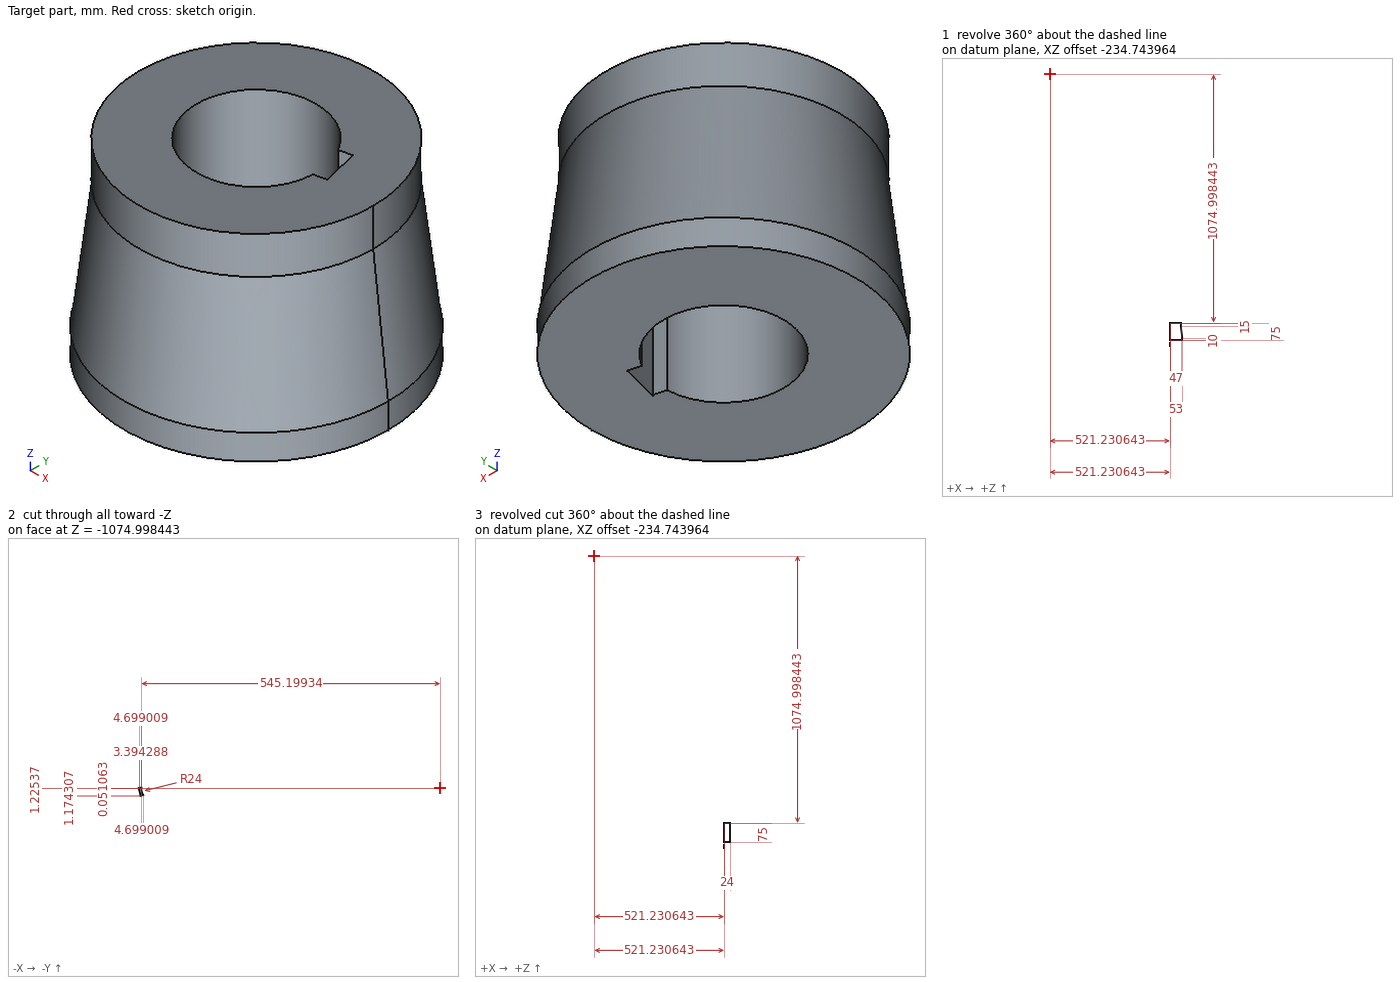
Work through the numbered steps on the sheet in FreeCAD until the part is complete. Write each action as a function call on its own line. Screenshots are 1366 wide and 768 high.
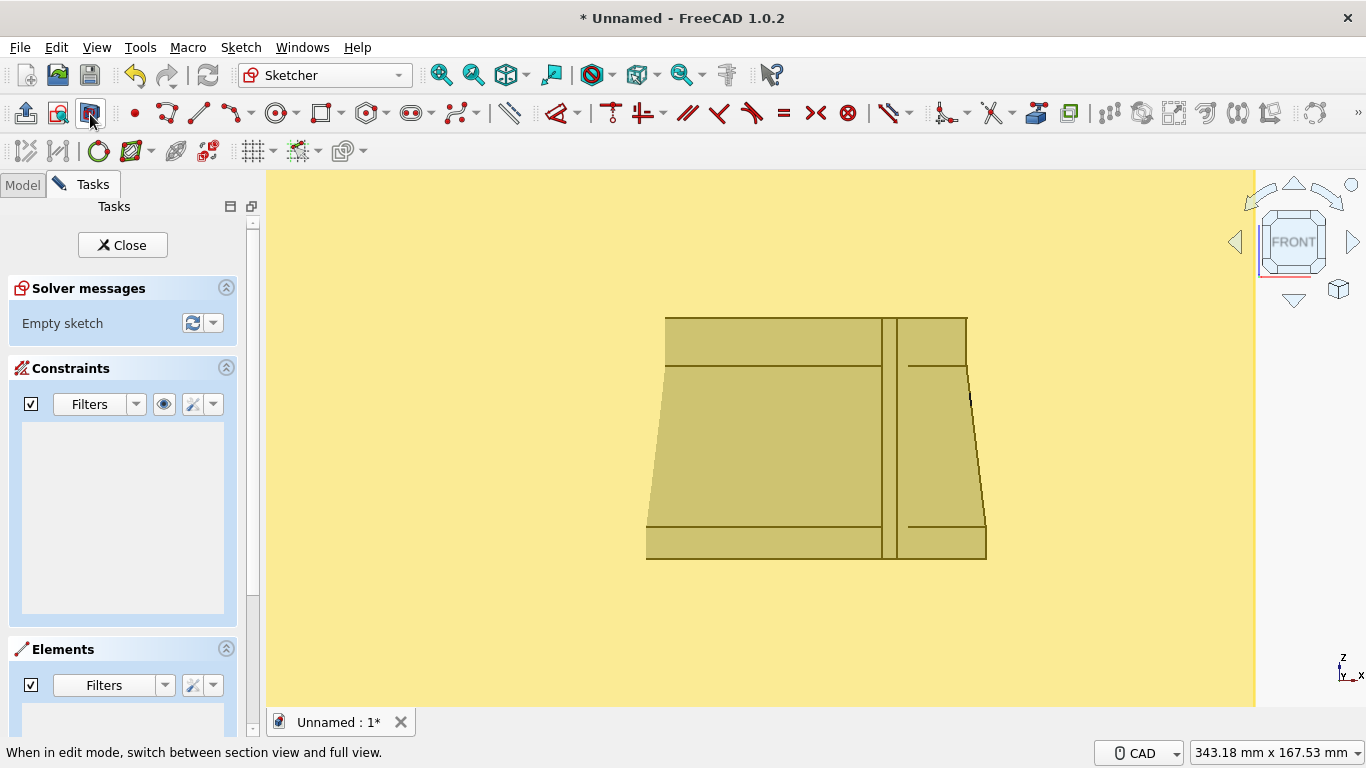
scroll(294, 221, down, 1)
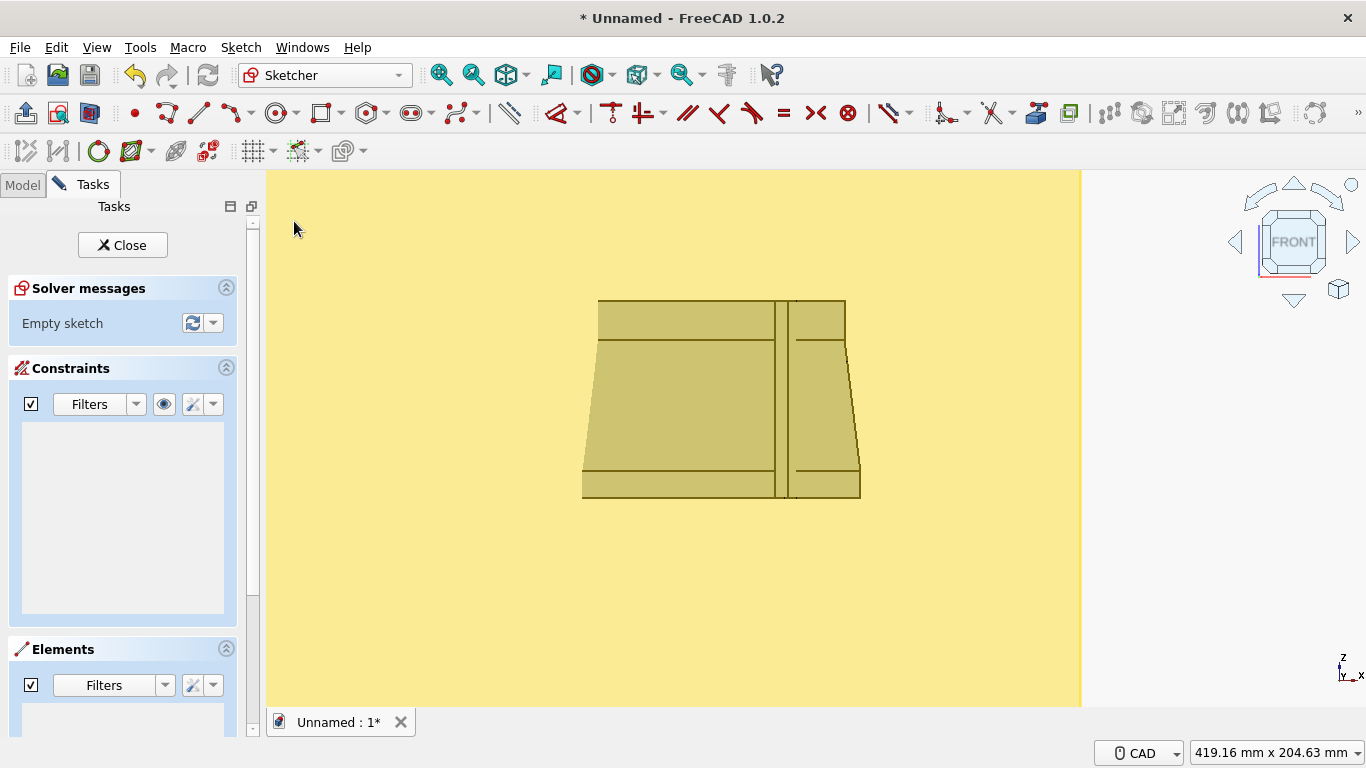
click(322, 114)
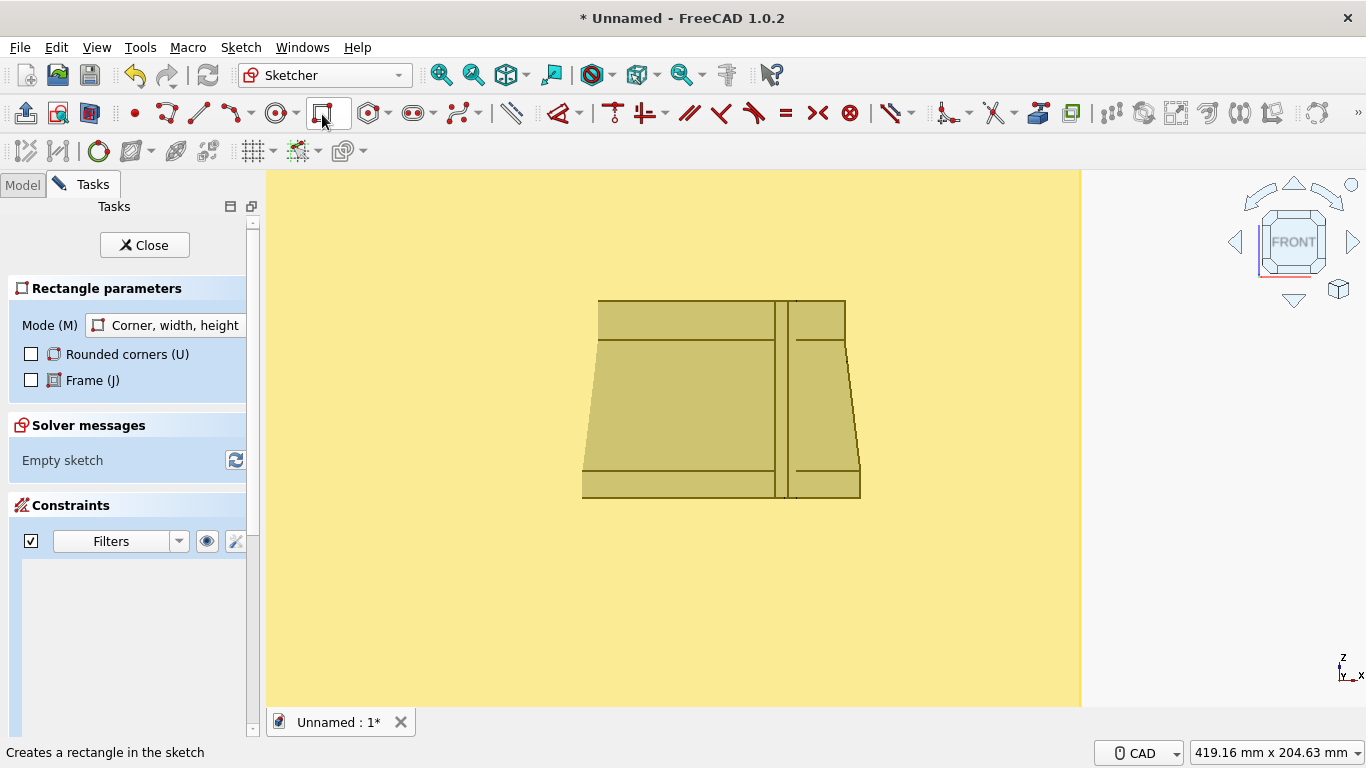
click(721, 301)
move(784, 498)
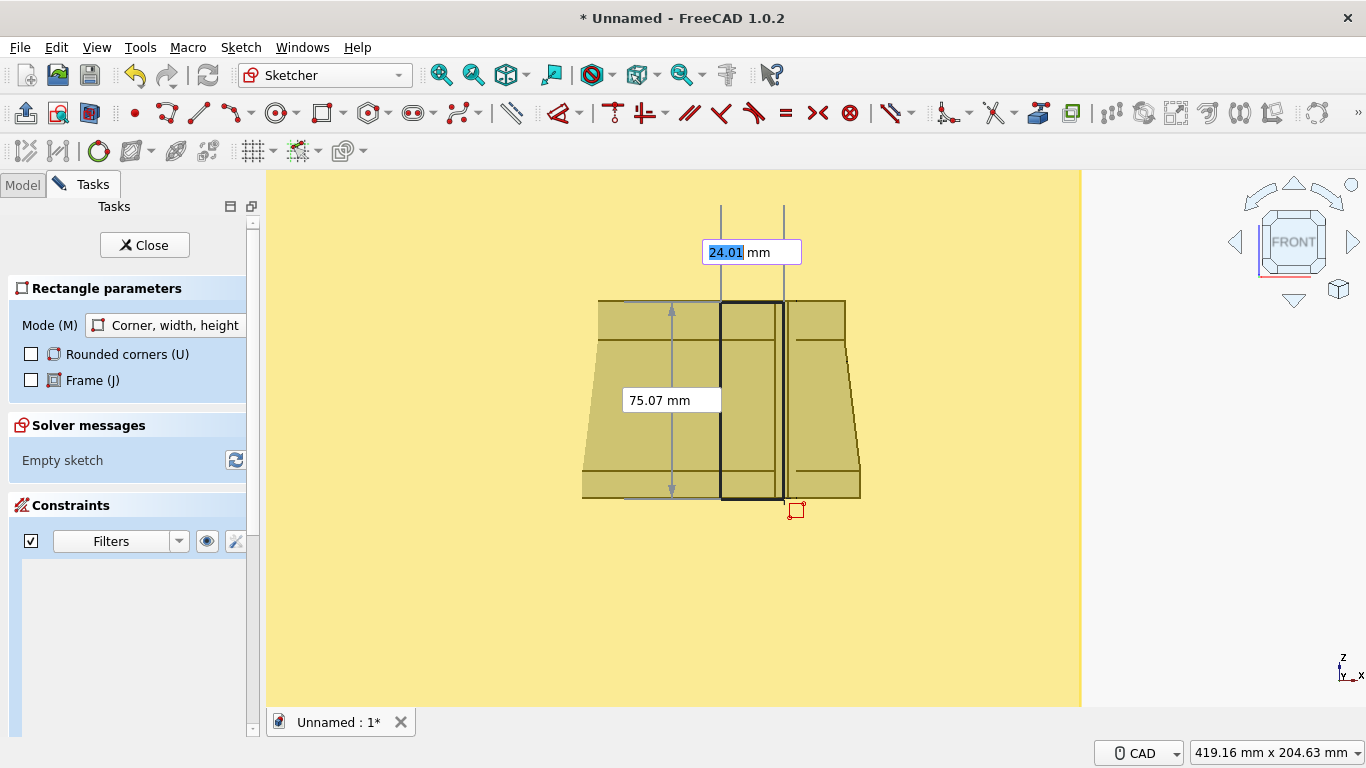
text(24)
key(Tab)
text(75)
key(Return)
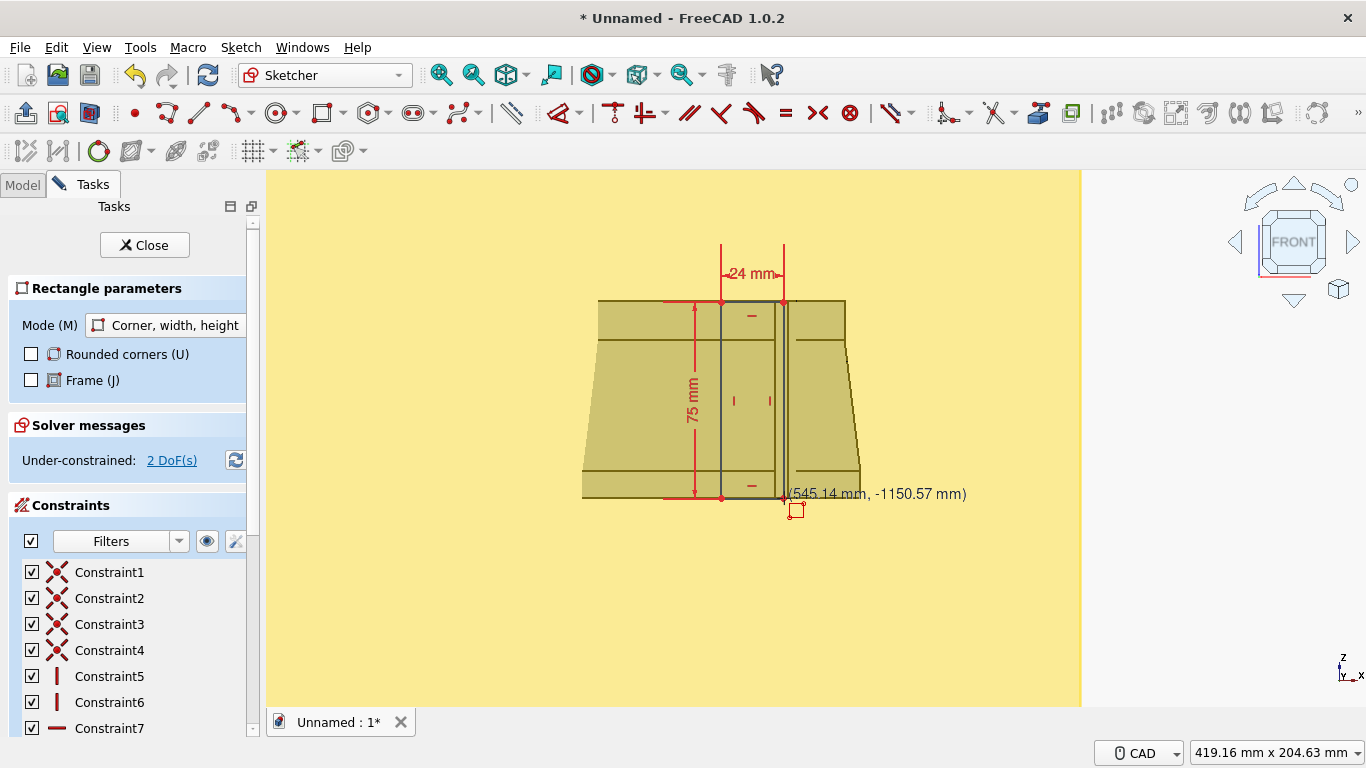
click(200, 114)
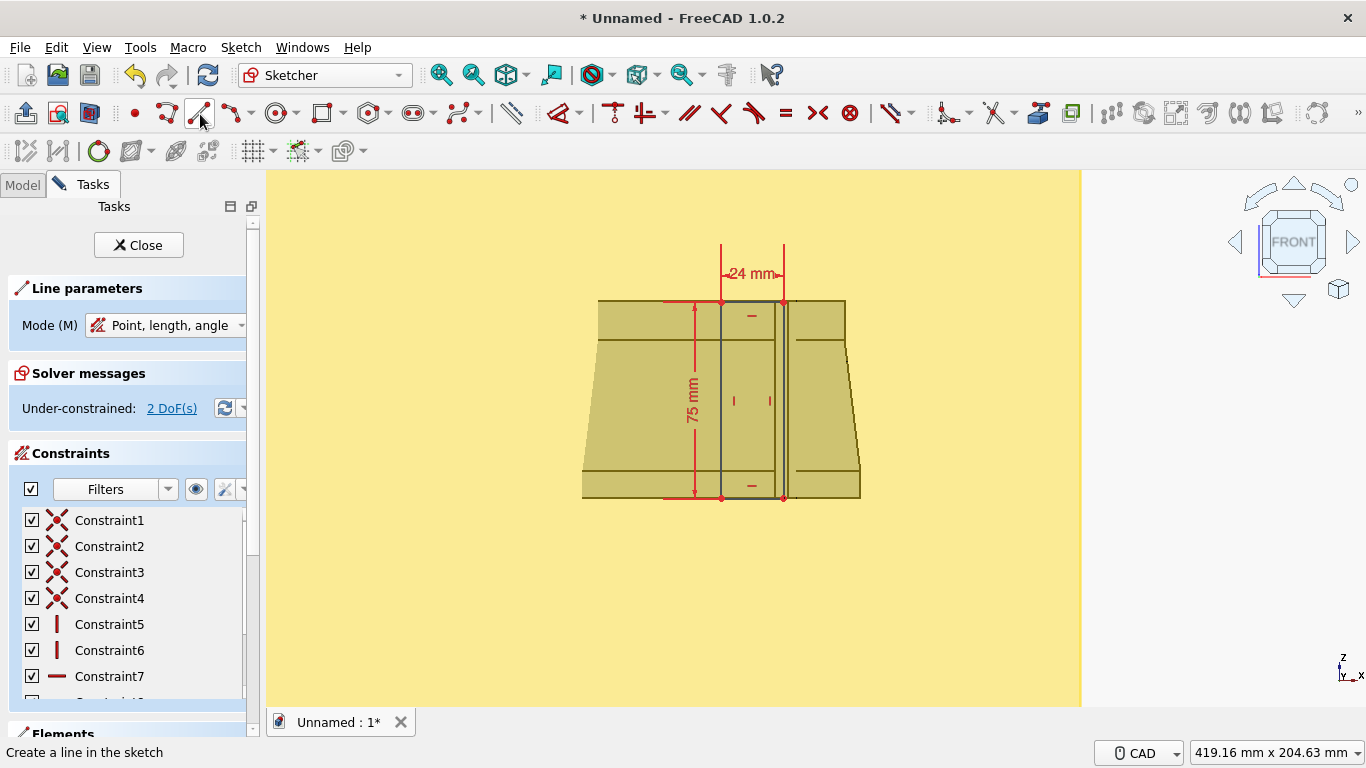
click(721, 517)
click(721, 576)
key(Escape)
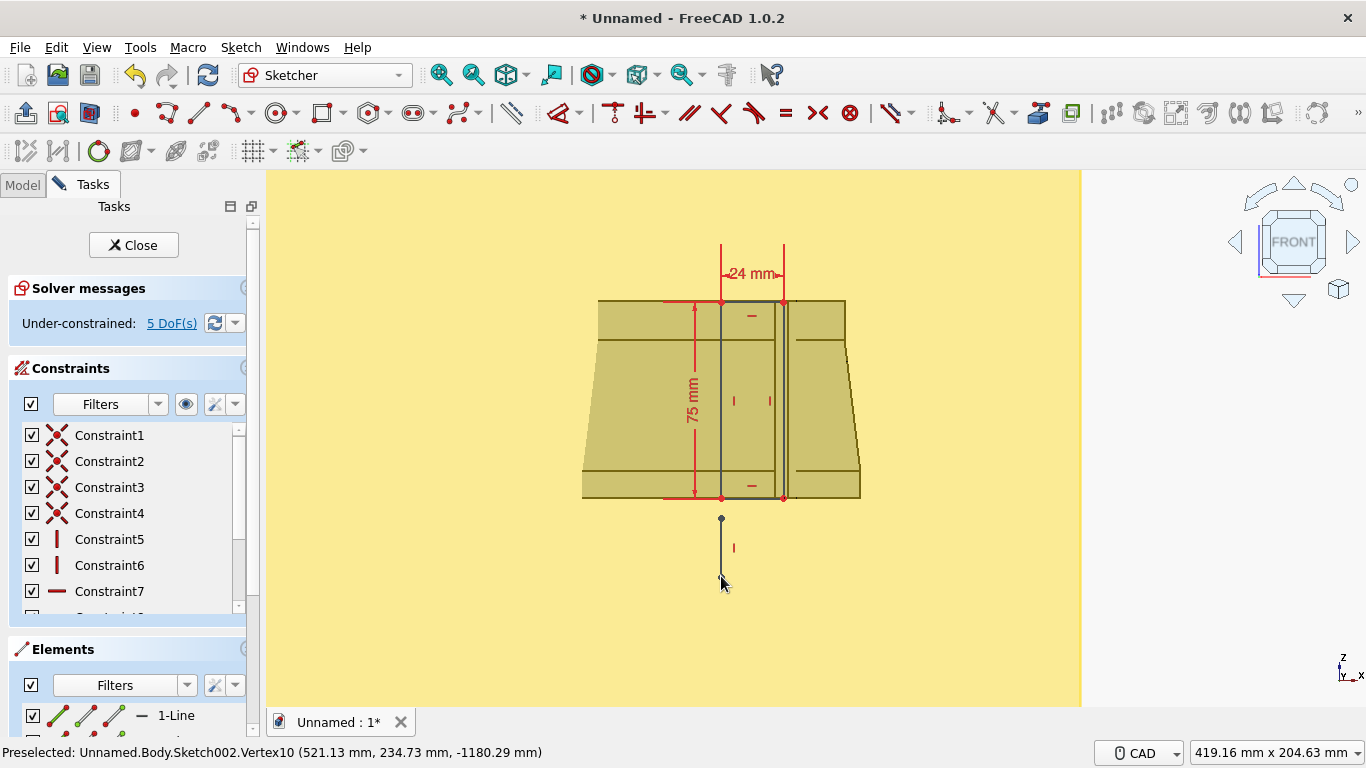
click(721, 536)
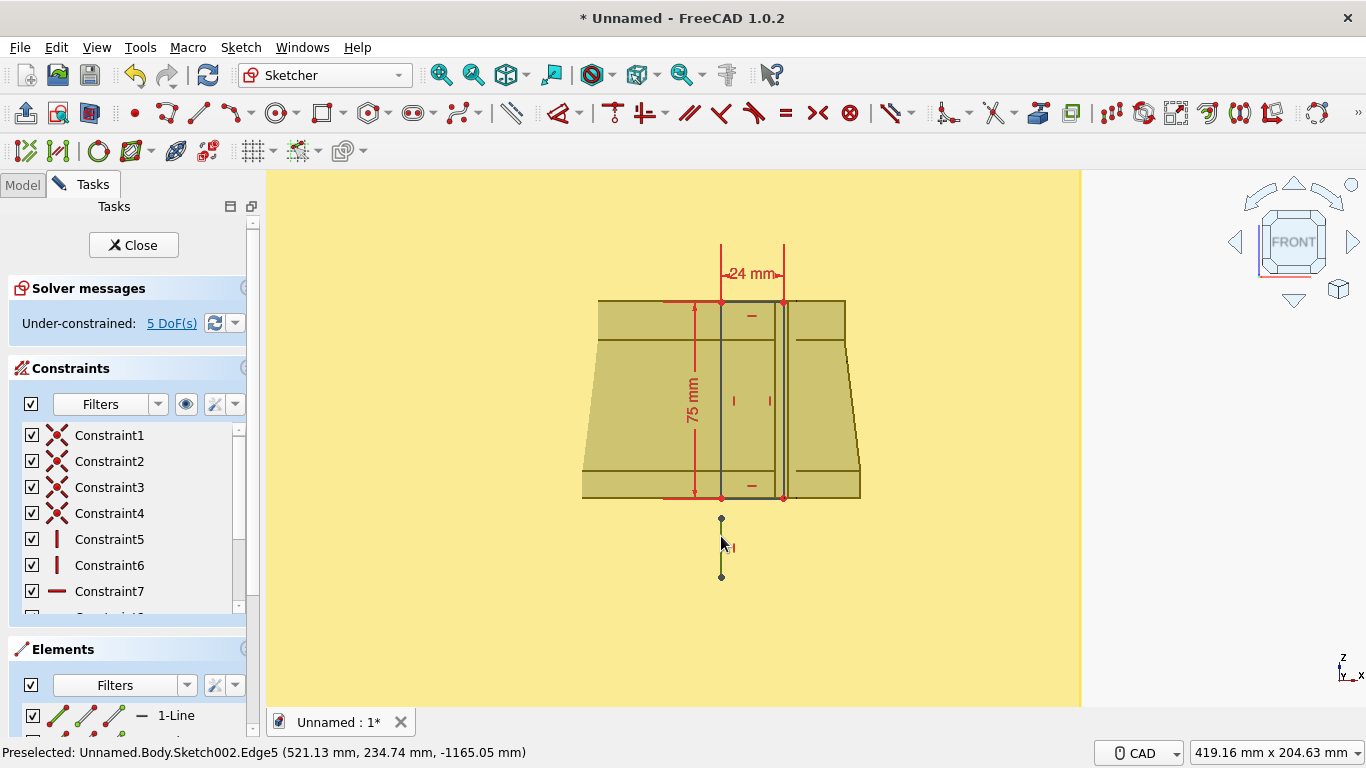
click(512, 114)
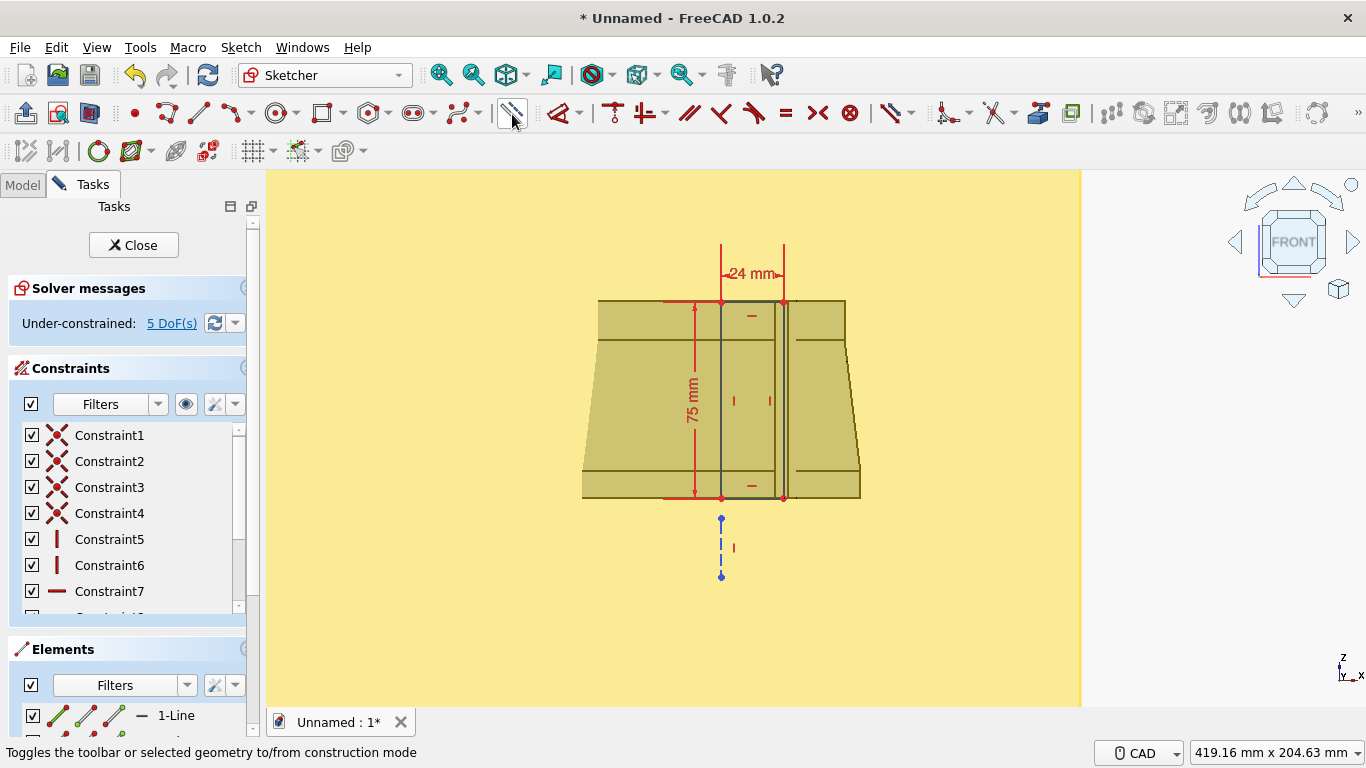
click(558, 114)